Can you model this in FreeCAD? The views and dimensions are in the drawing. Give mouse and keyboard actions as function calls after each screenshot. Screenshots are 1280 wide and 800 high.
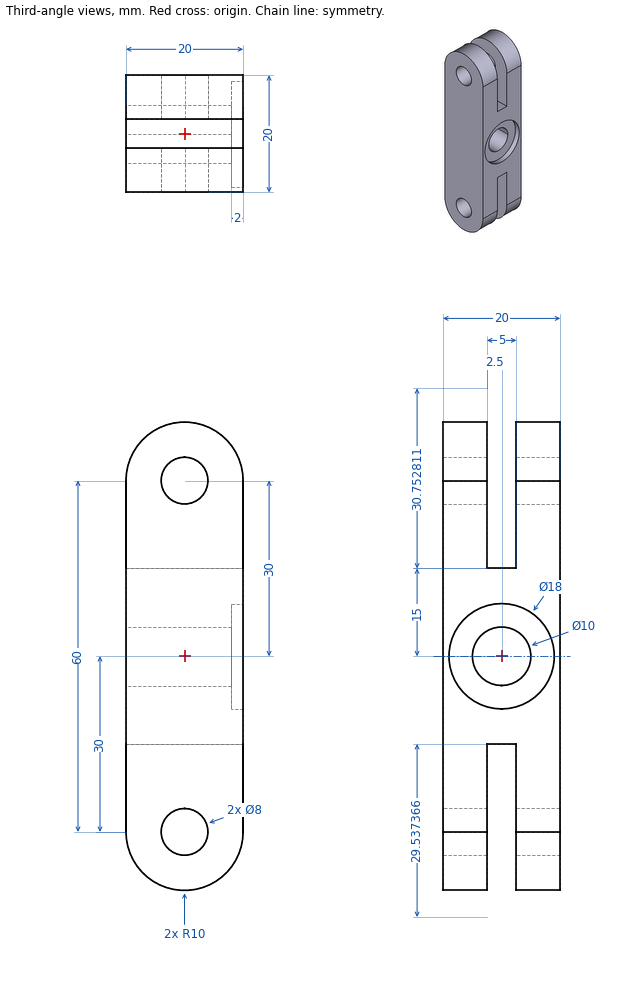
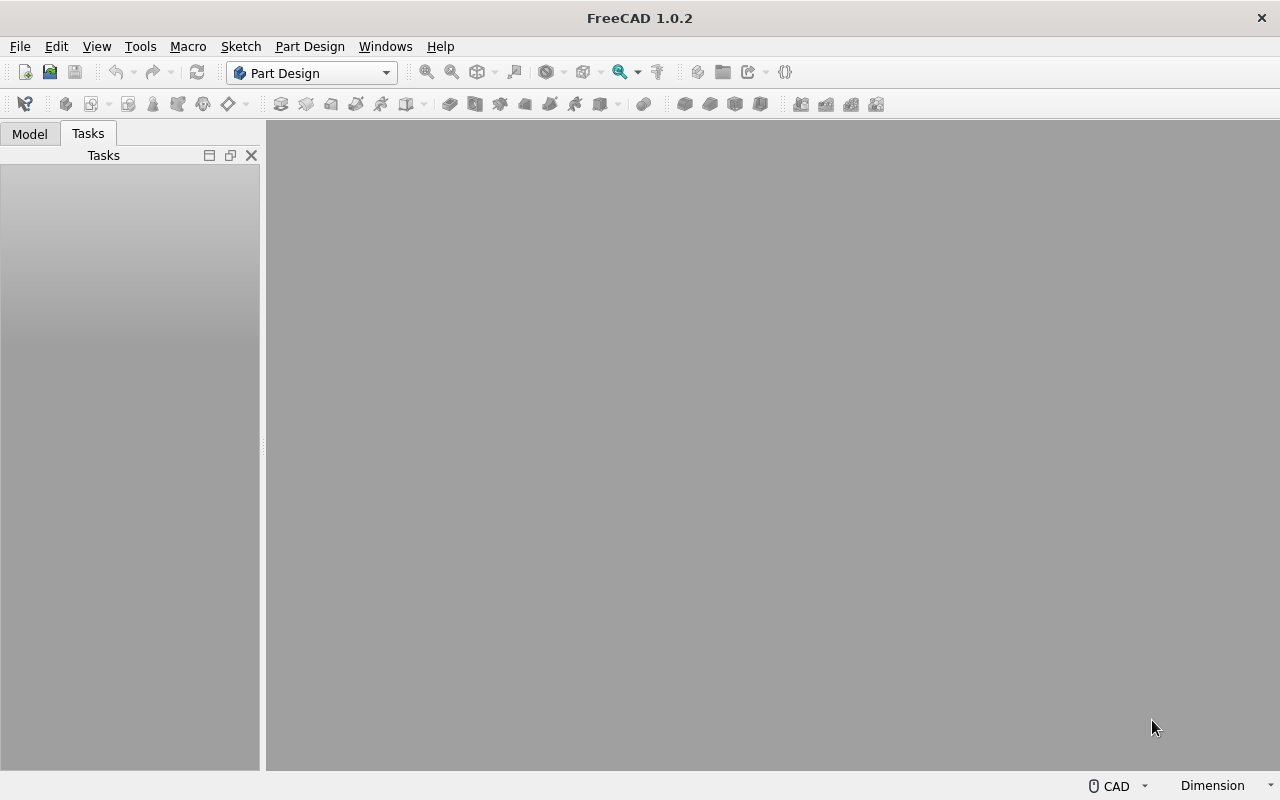
key(ctrl+n)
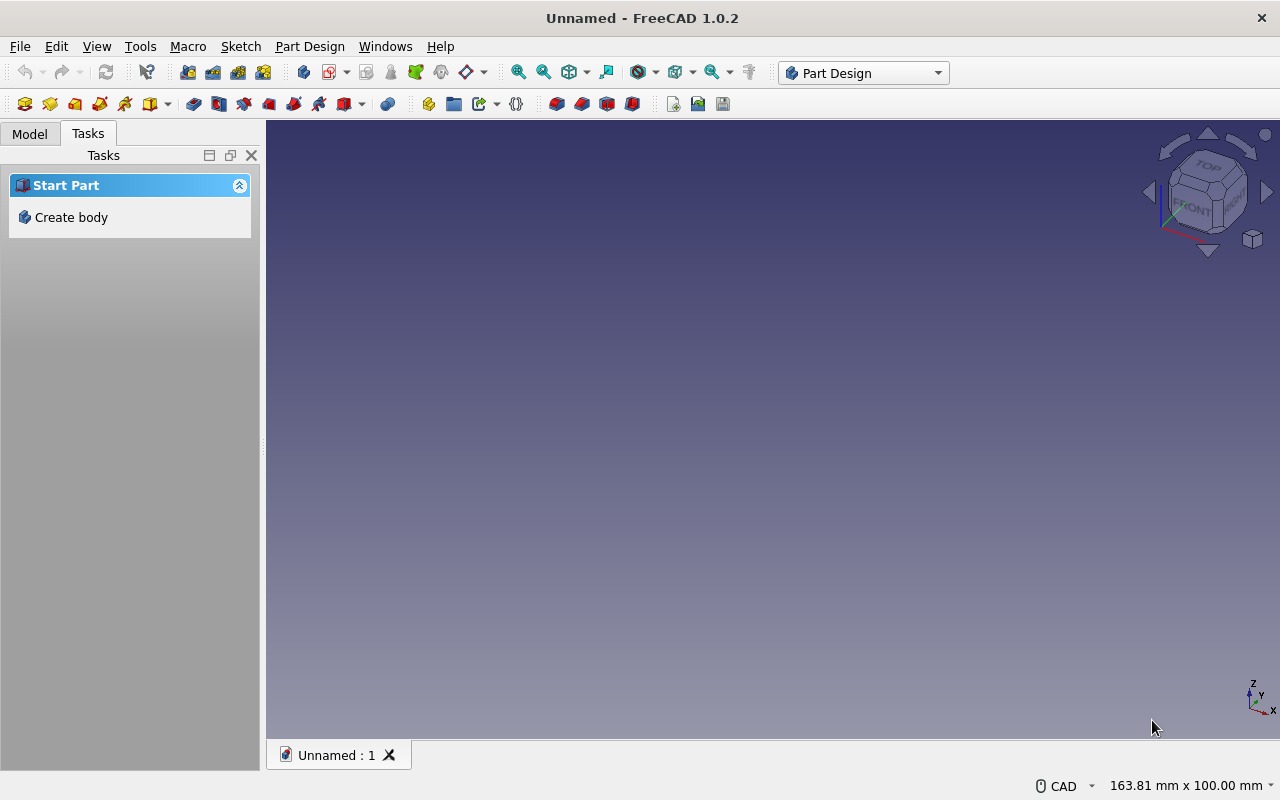
click(328, 72)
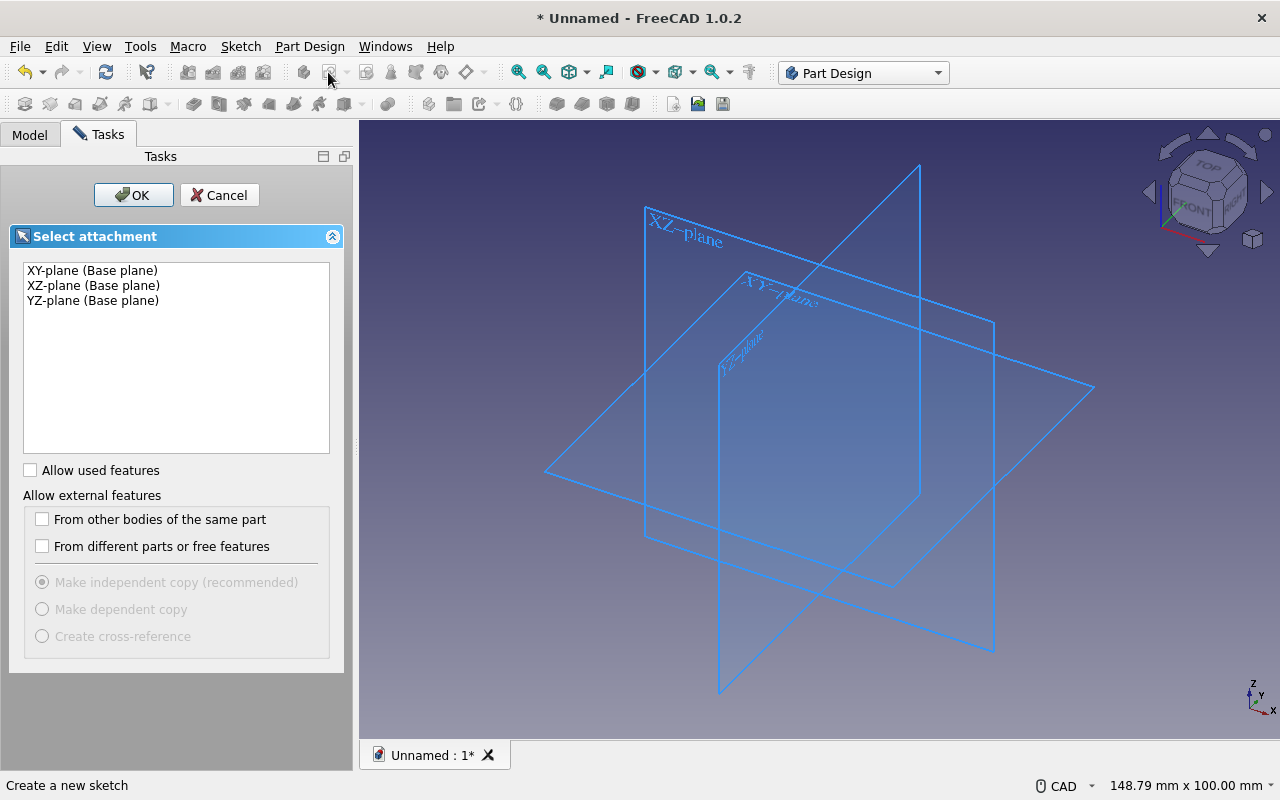
click(84, 286)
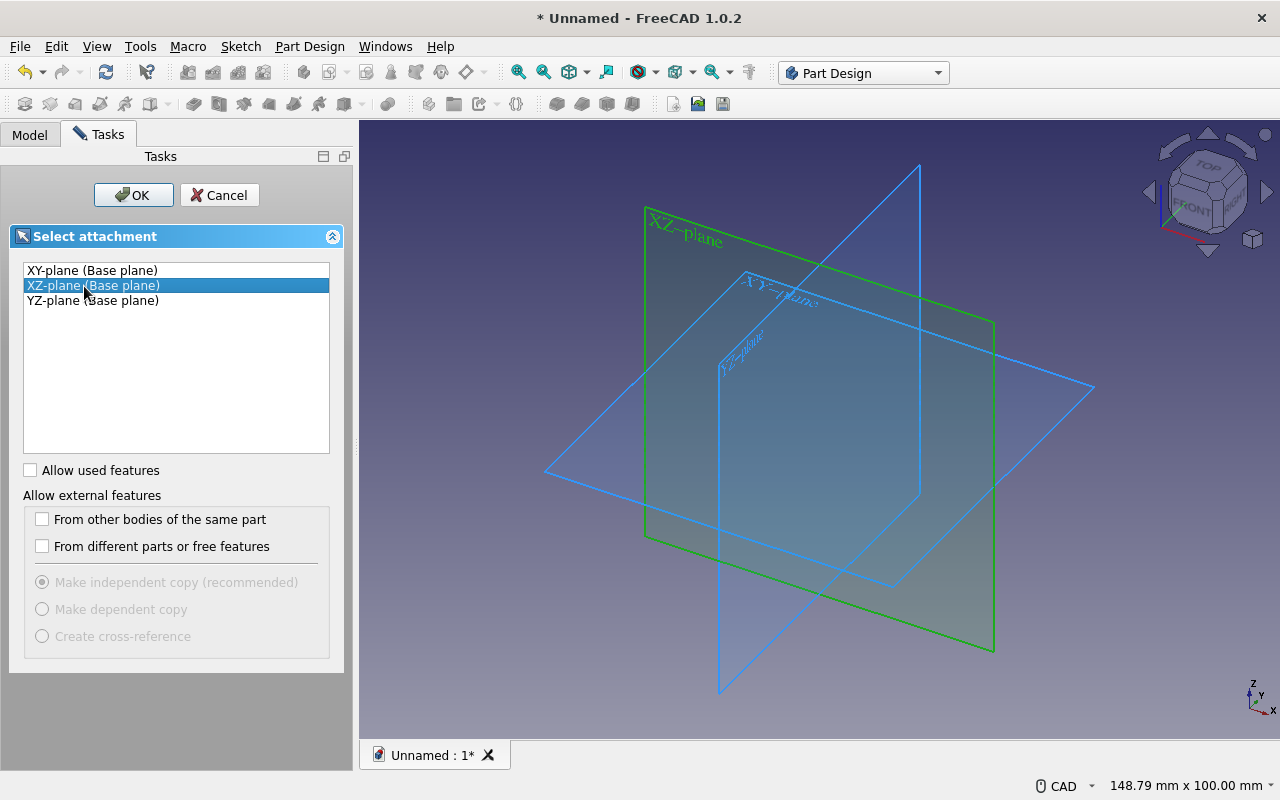
click(134, 195)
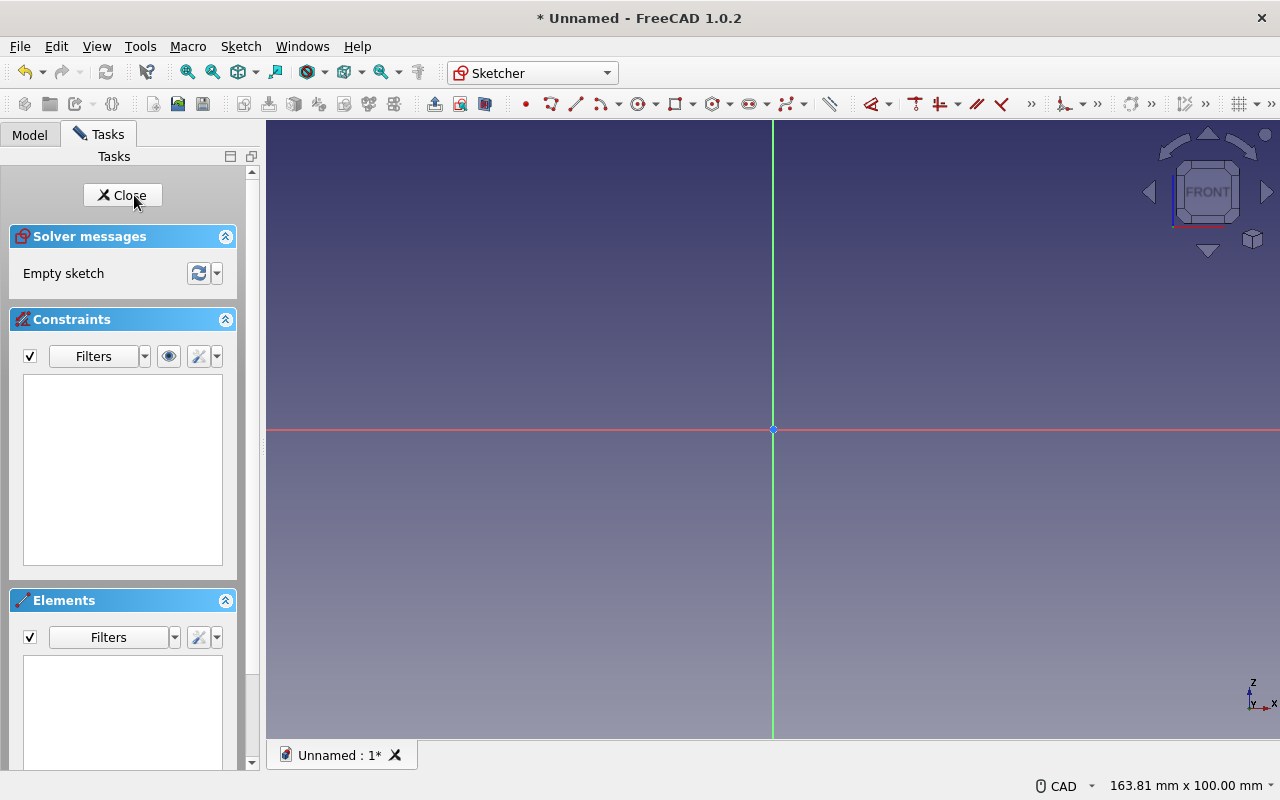
key(g)
key(s)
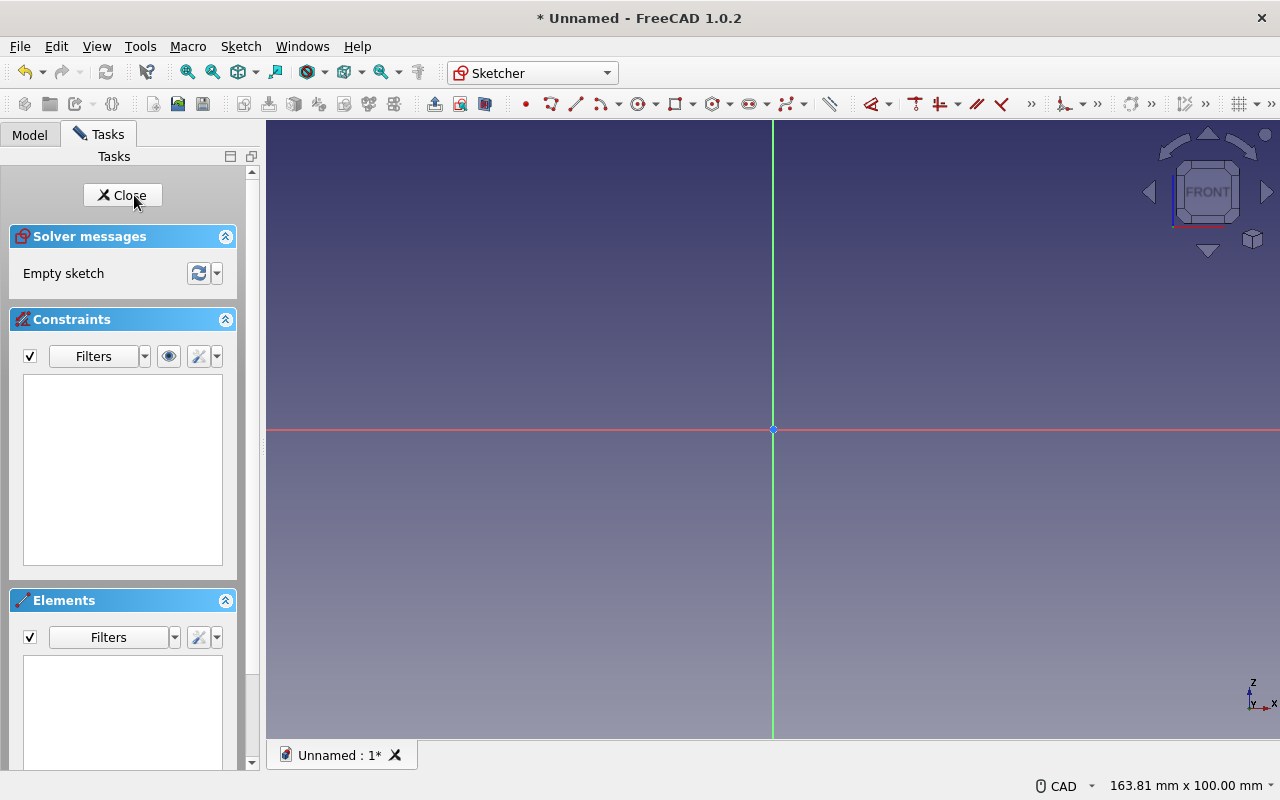
click(773, 615)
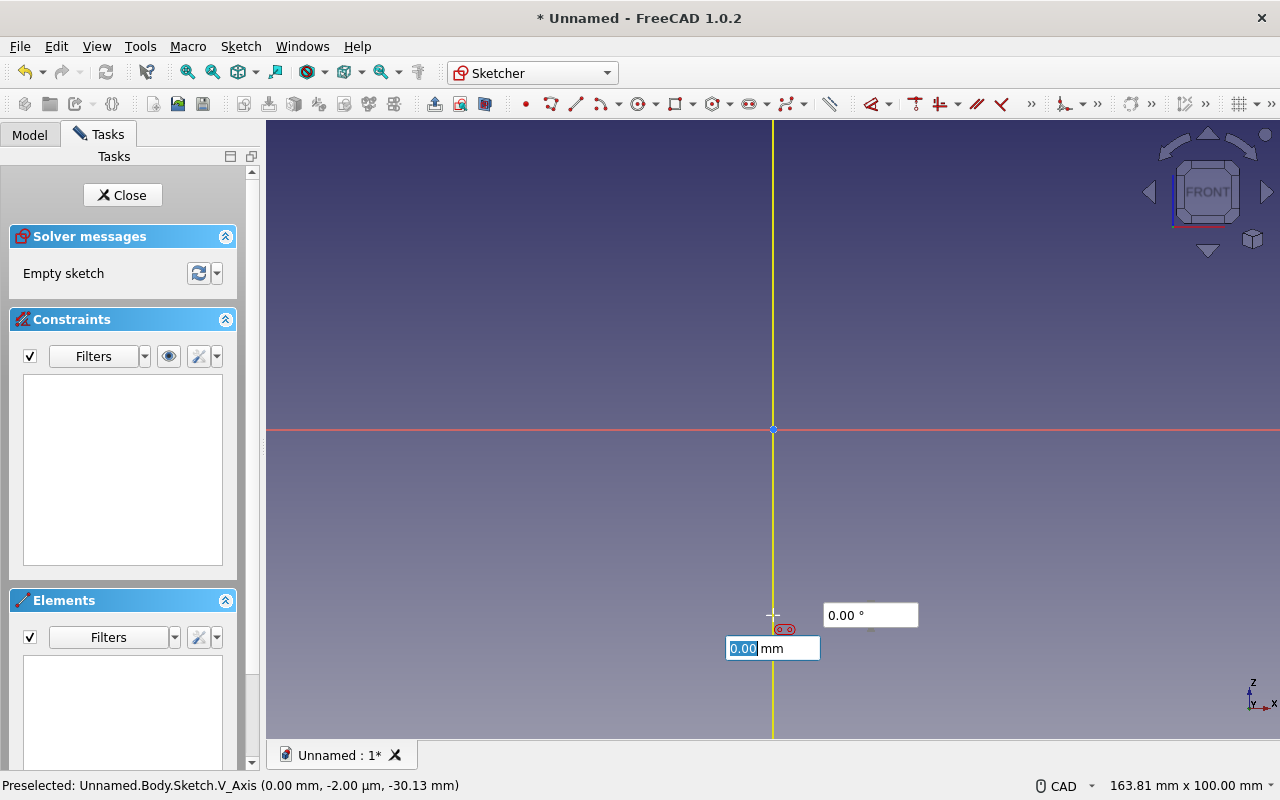
click(782, 244)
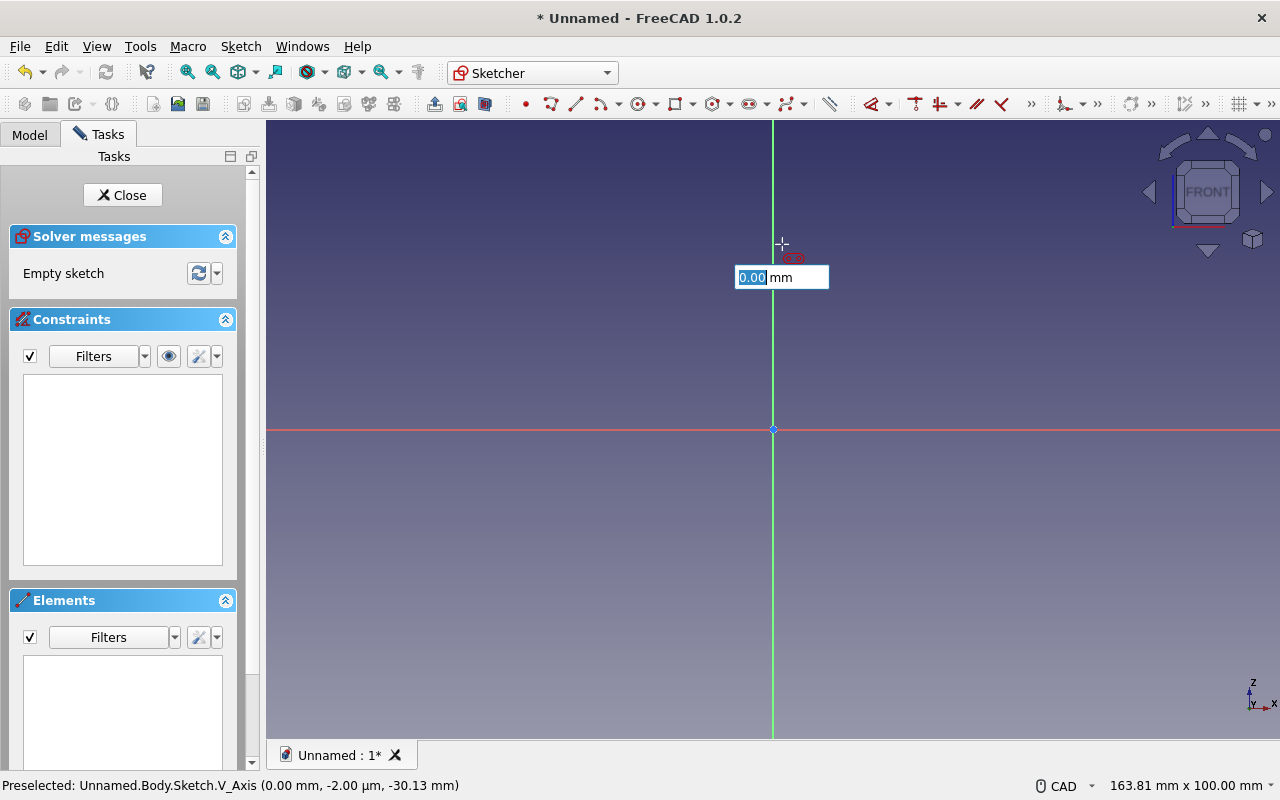
click(835, 374)
key(Escape)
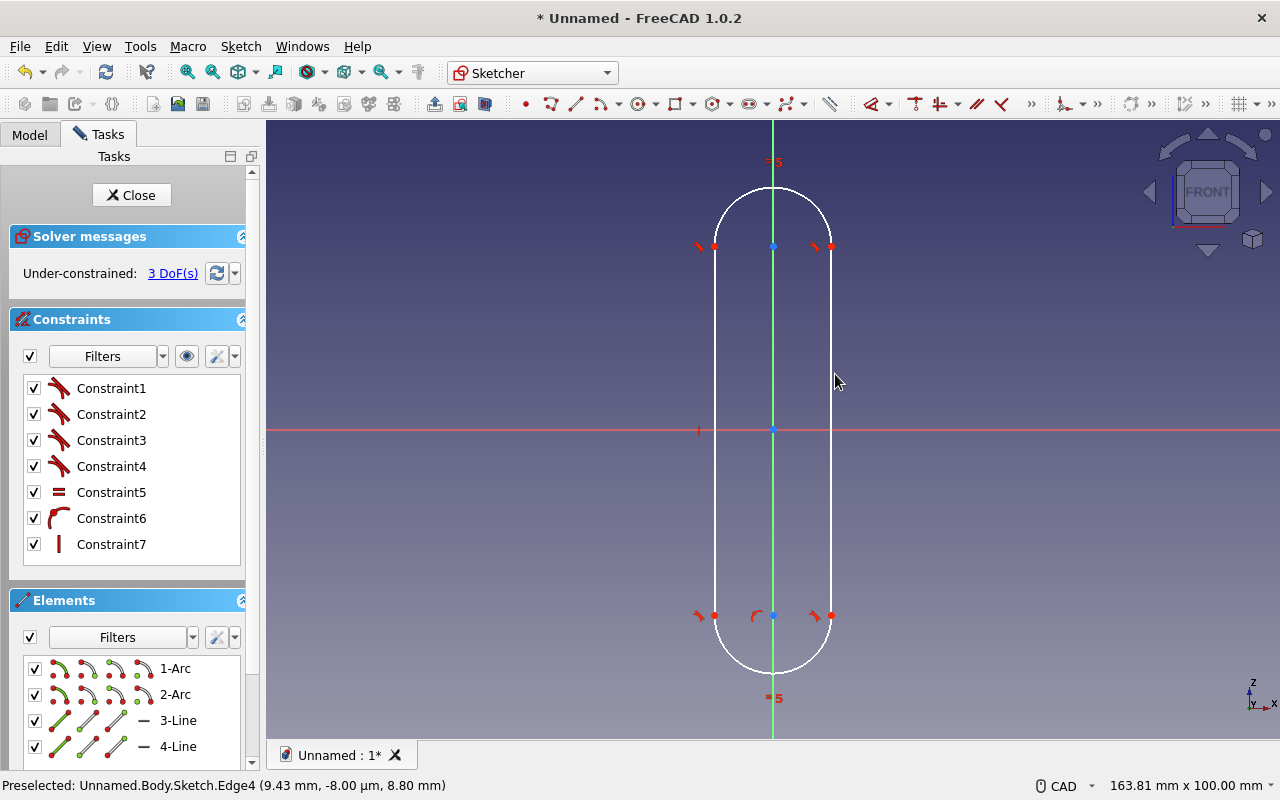
key(d)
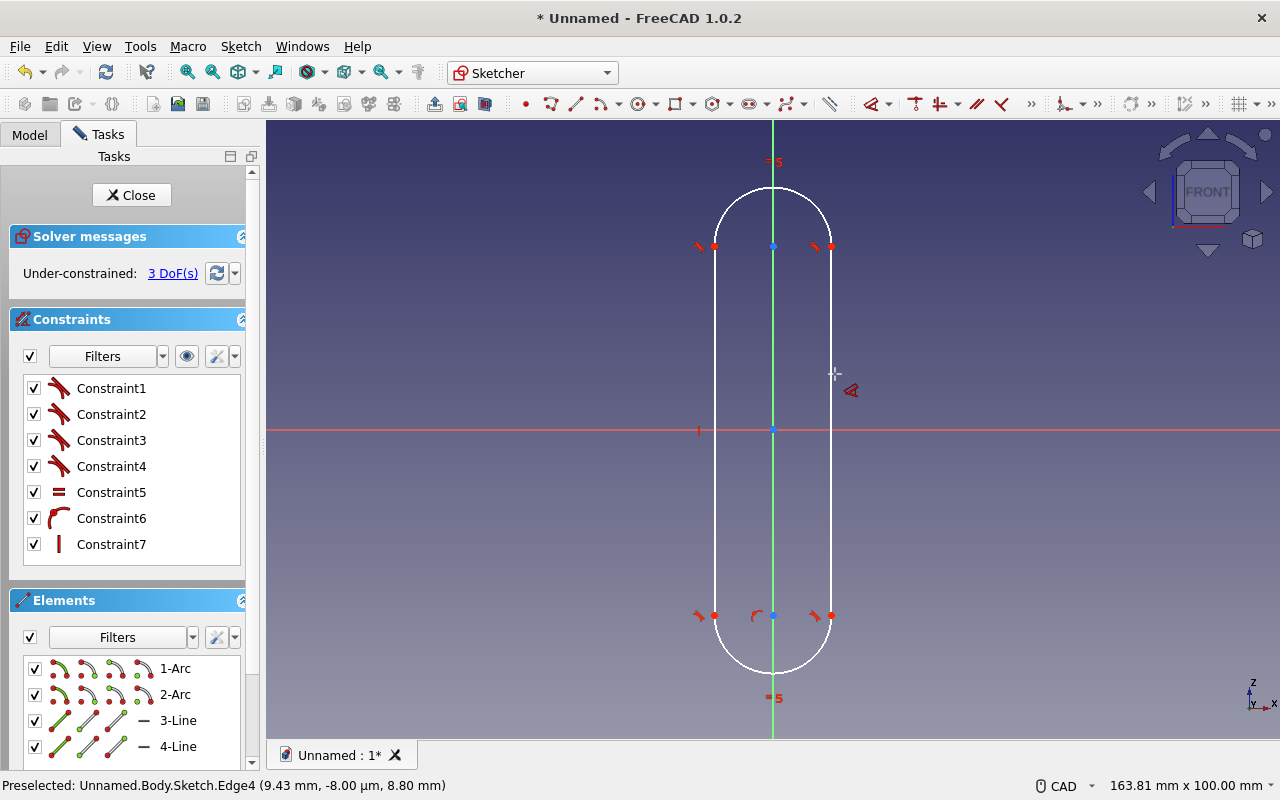
click(739, 662)
click(720, 688)